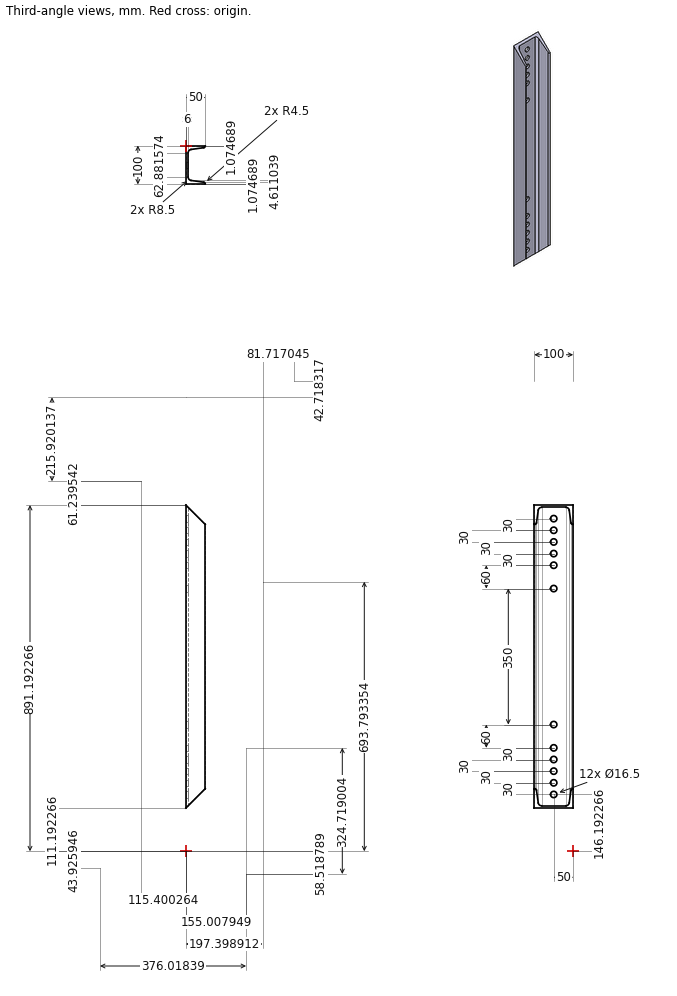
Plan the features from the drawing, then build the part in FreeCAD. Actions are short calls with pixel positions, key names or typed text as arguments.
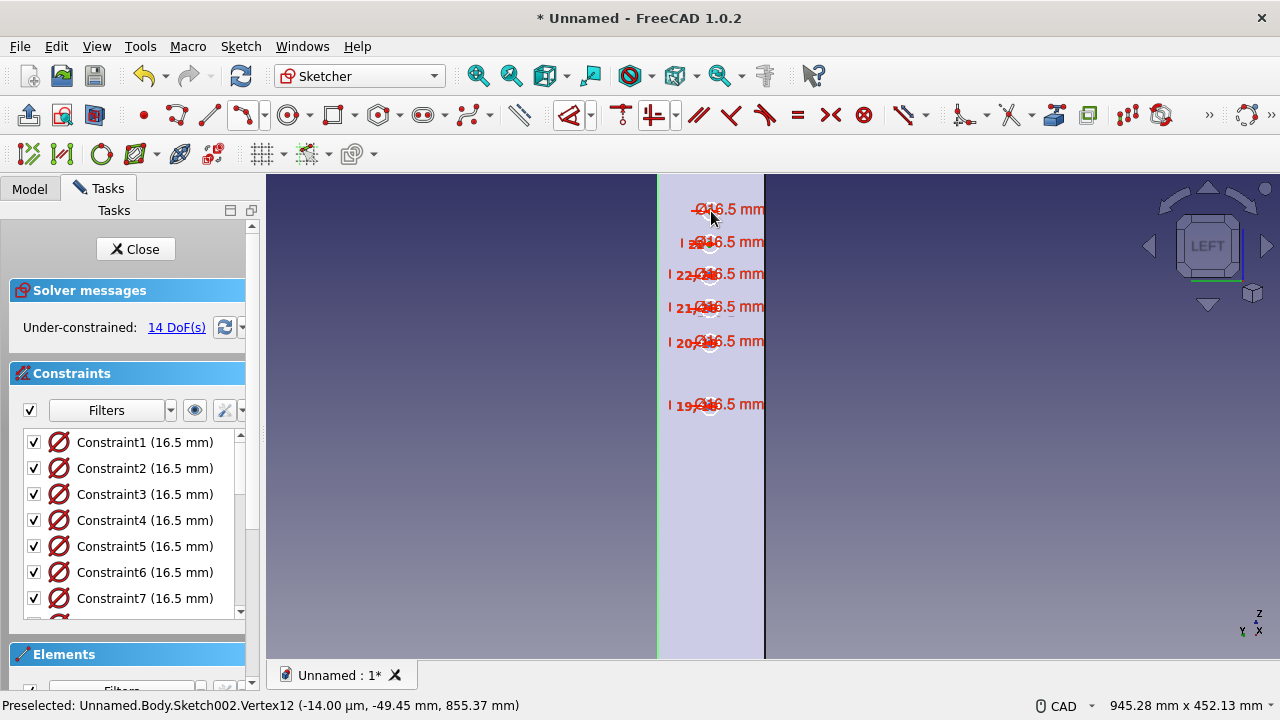
key(v)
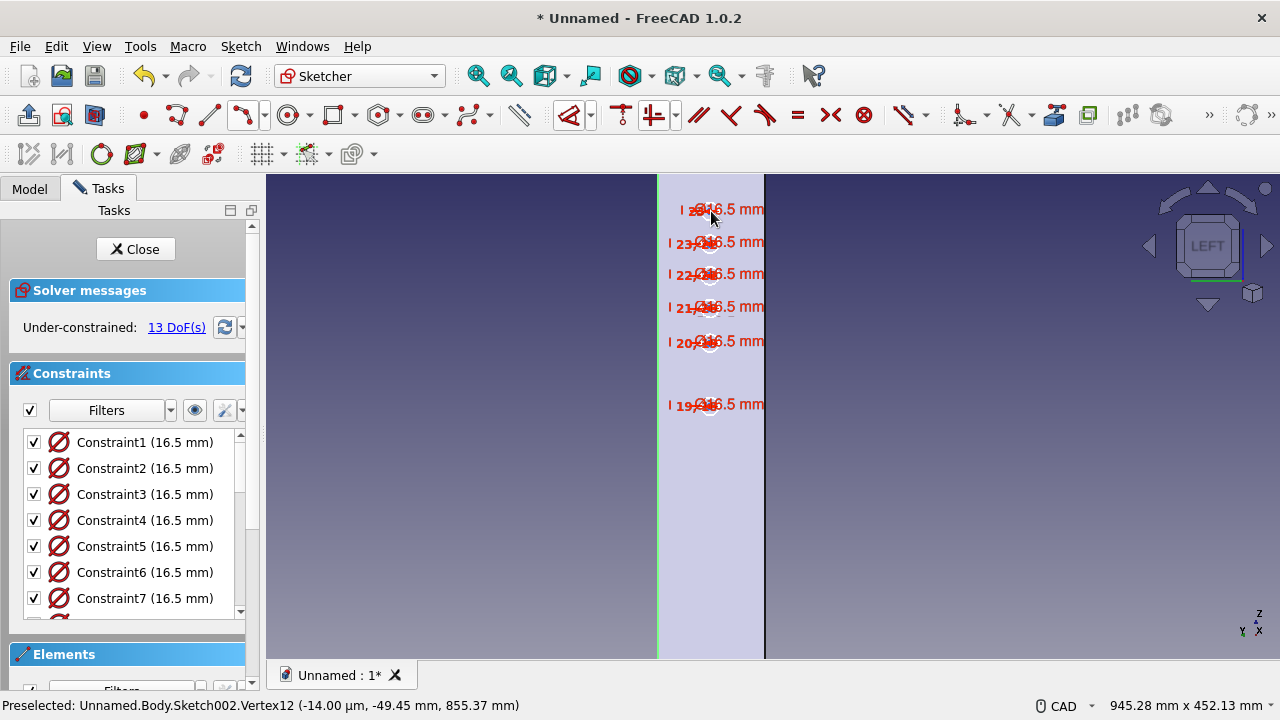
scroll(711, 309, down, 6)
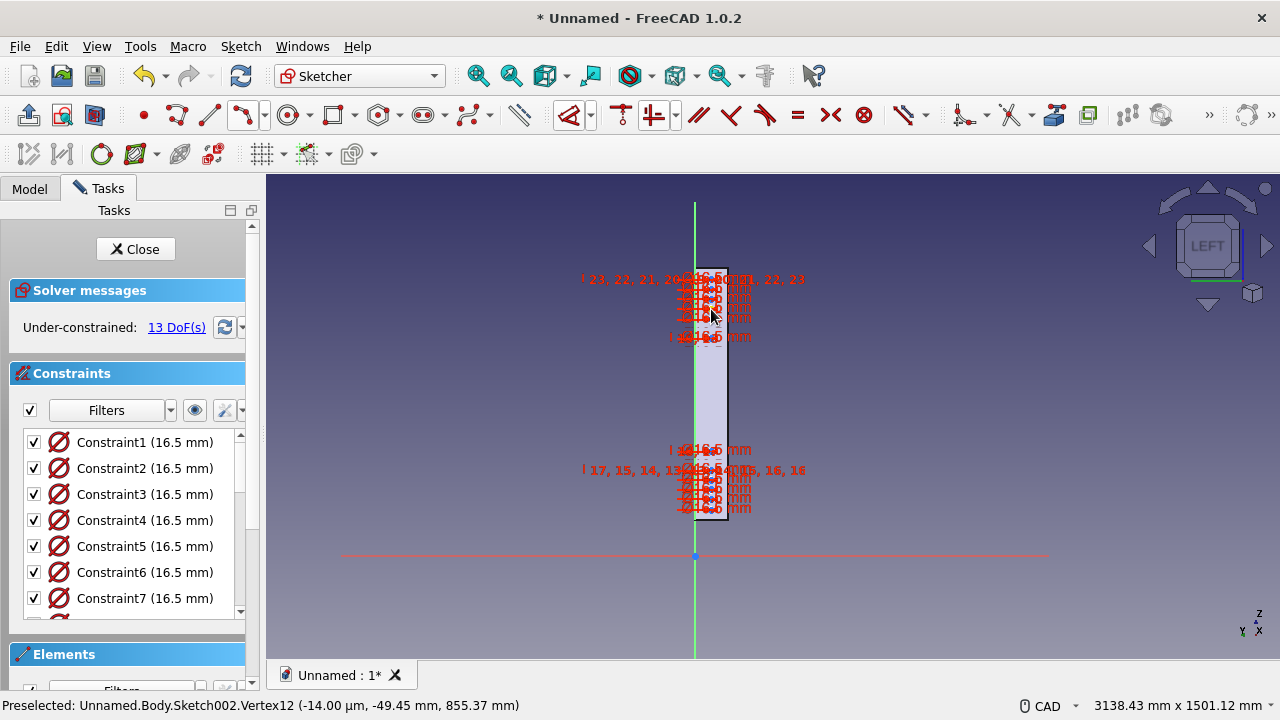
scroll(711, 510, up, 5)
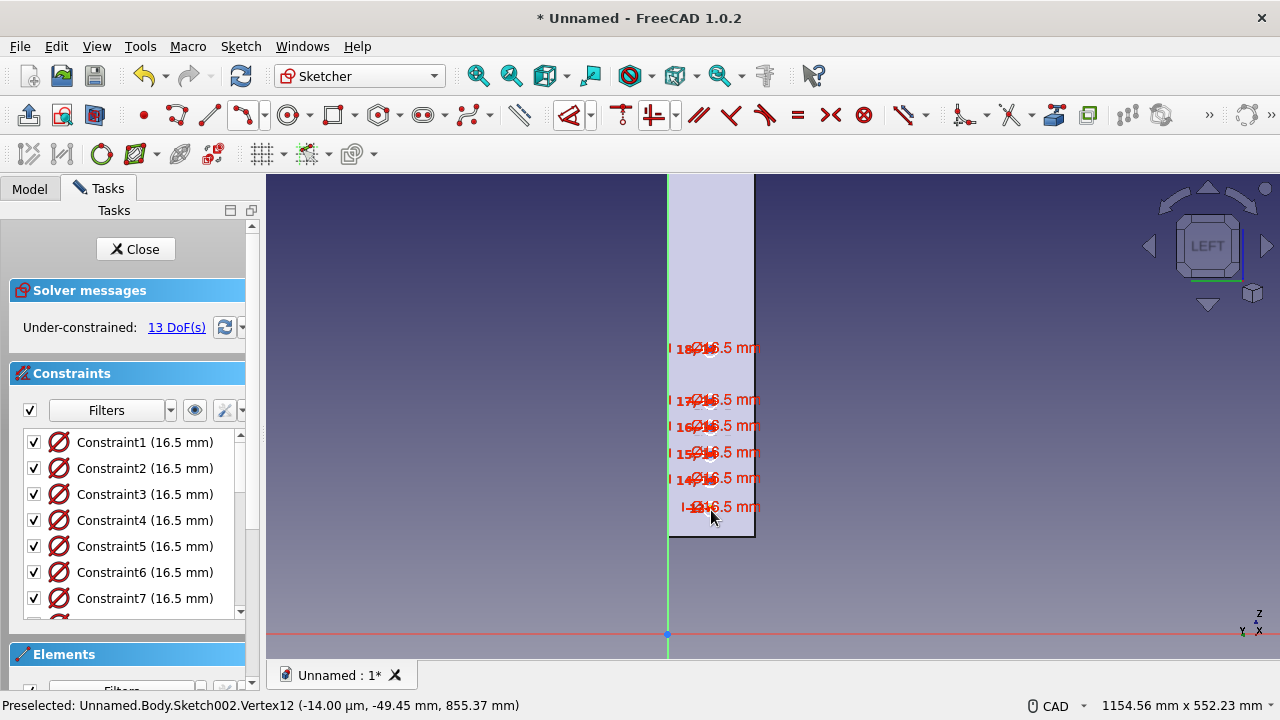
click(710, 509)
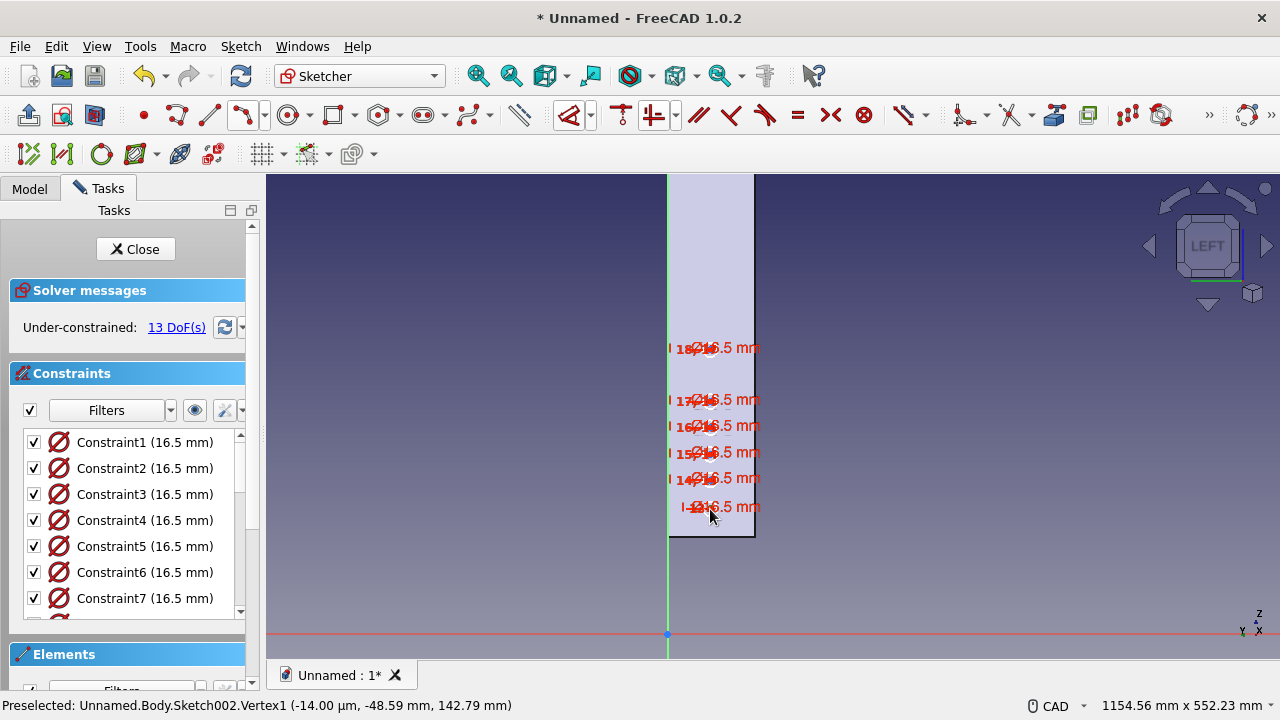
click(590, 116)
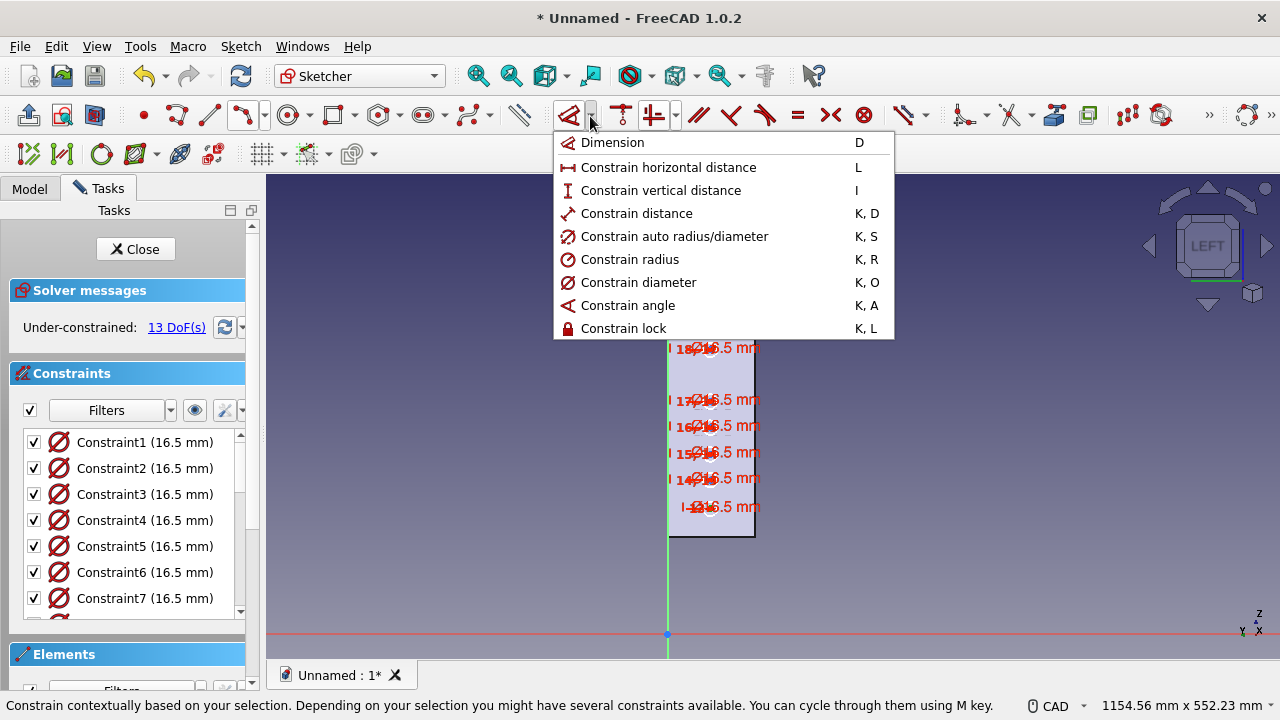
click(724, 168)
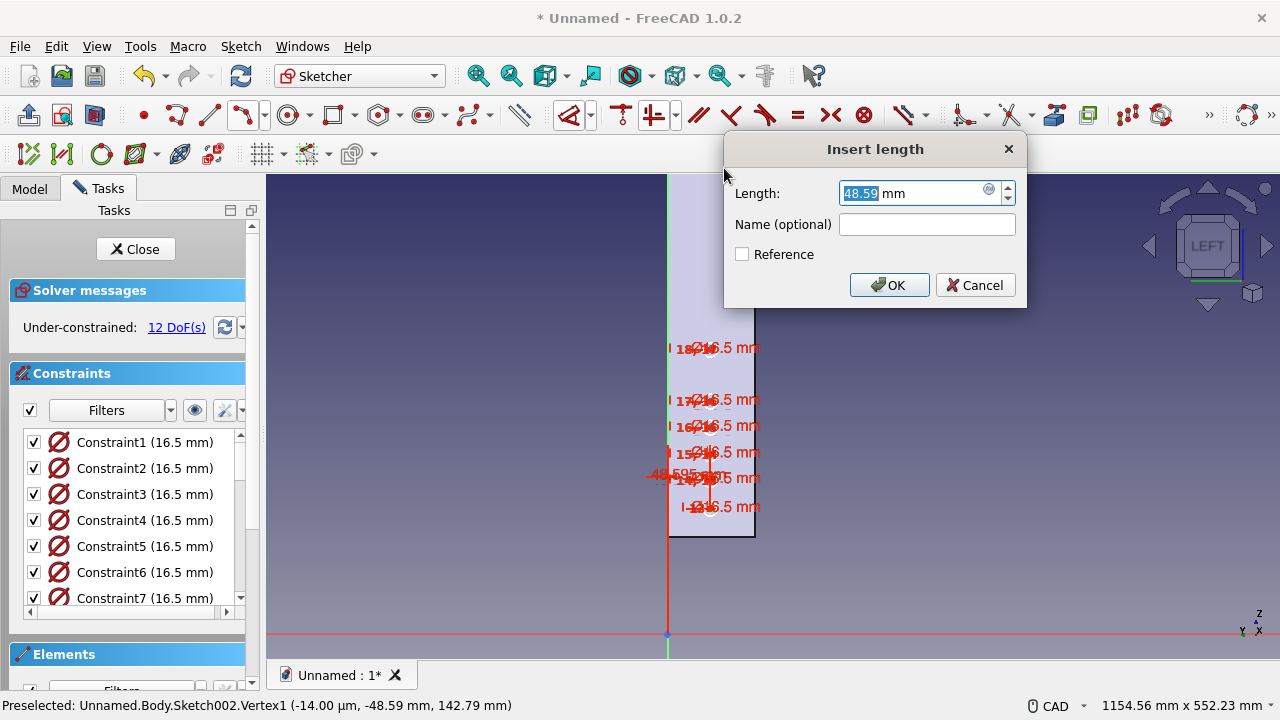
text(50)
key(Return)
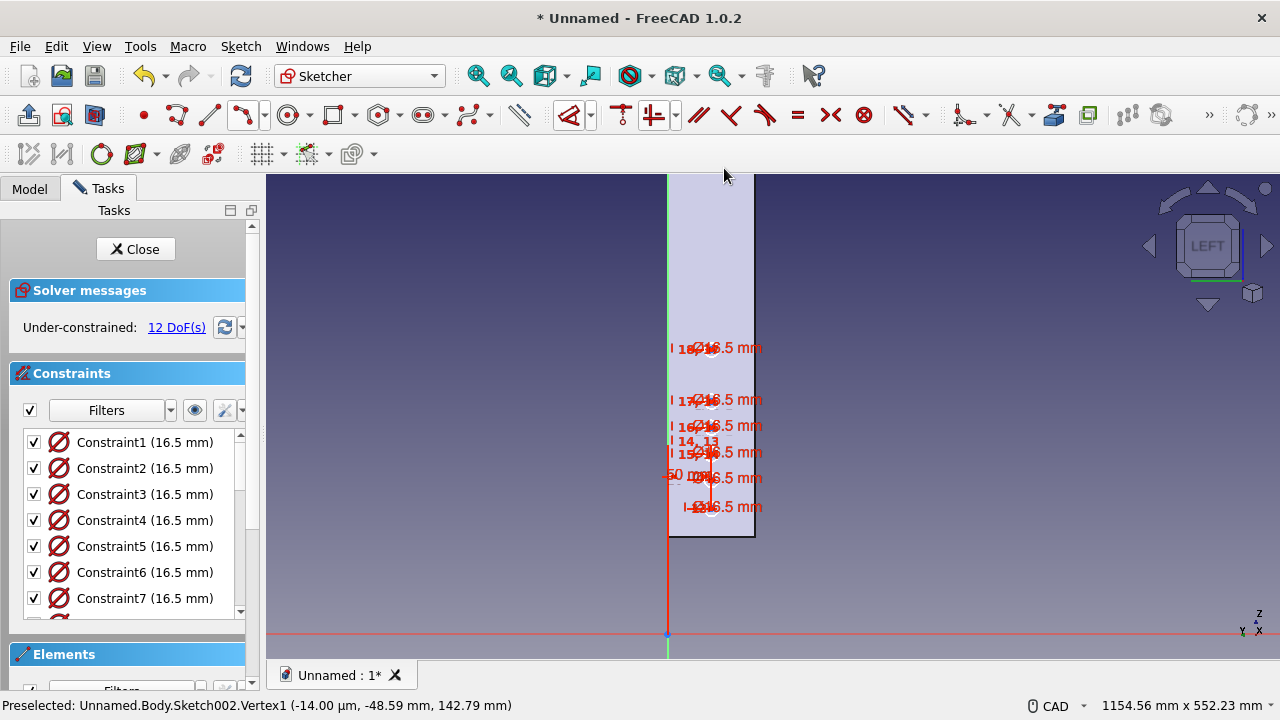
scroll(711, 509, up, 3)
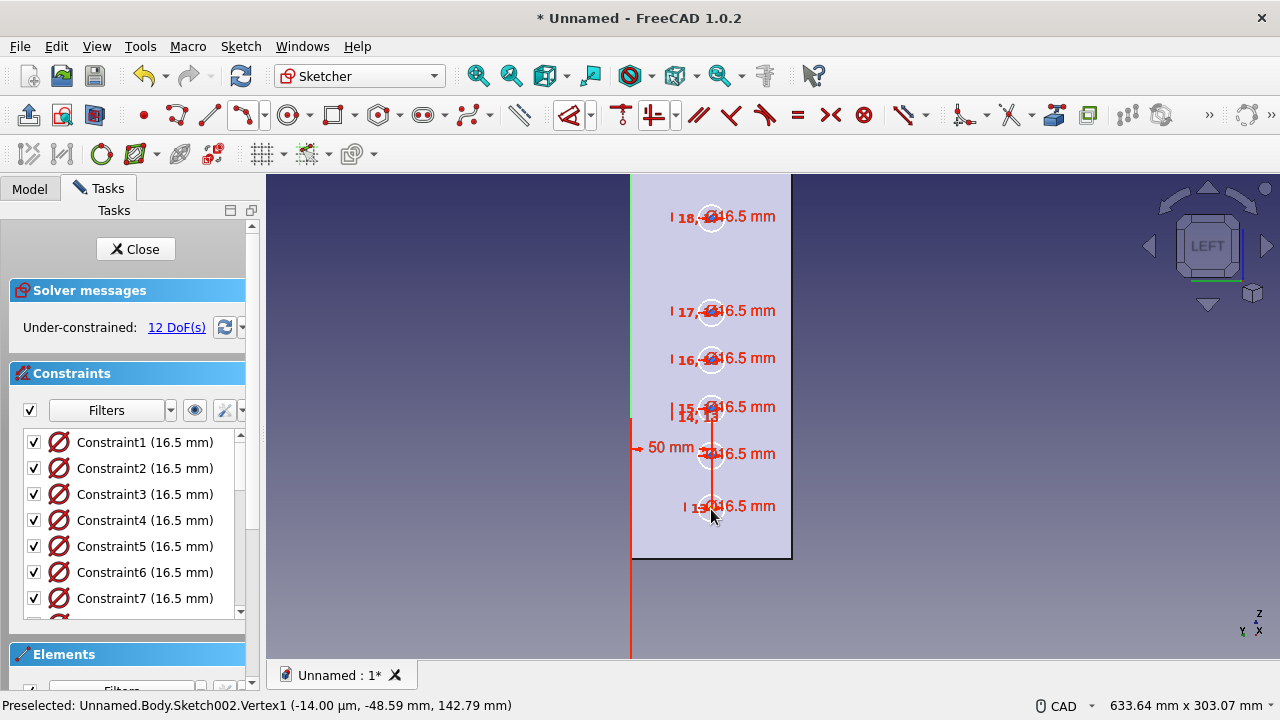
click(712, 508)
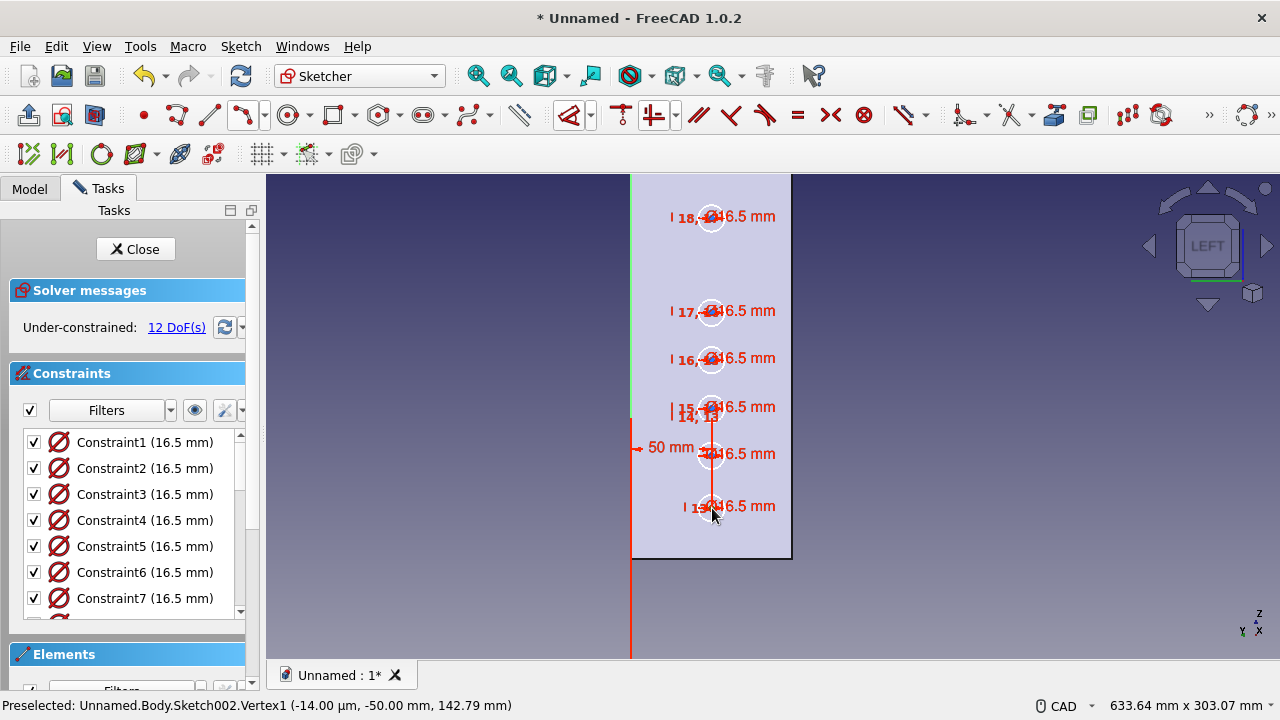
click(712, 456)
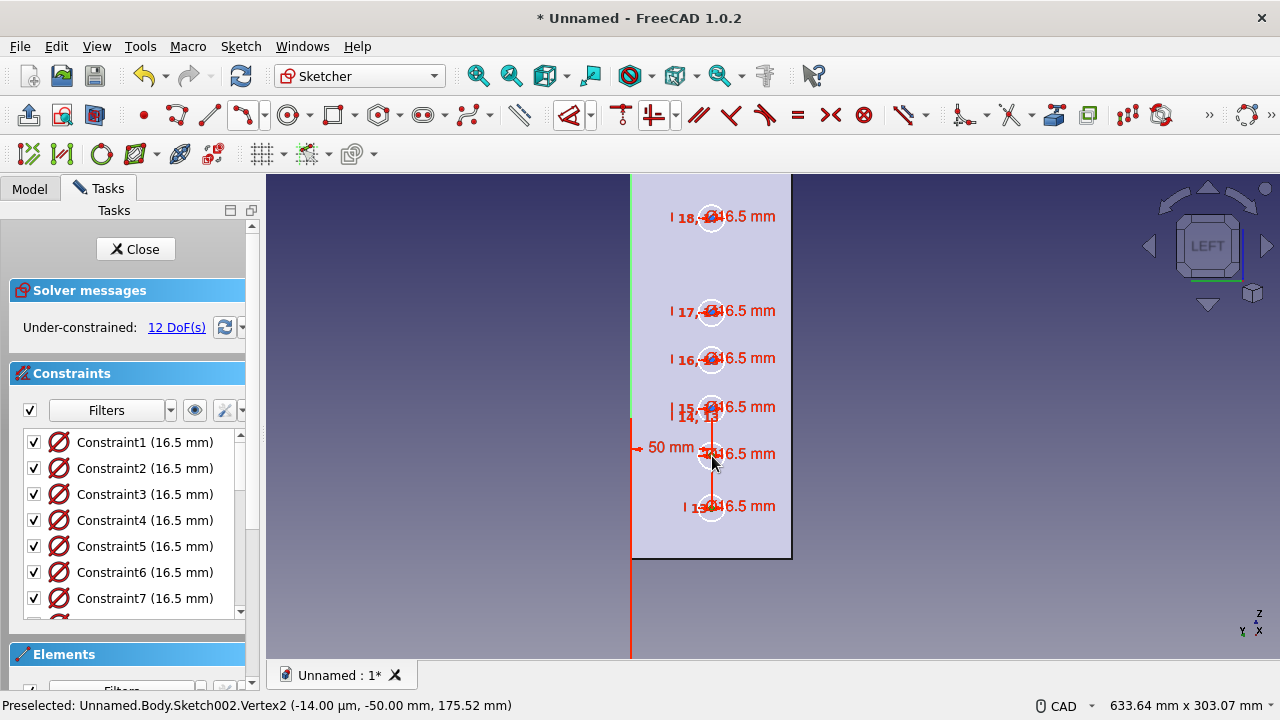
key(i)